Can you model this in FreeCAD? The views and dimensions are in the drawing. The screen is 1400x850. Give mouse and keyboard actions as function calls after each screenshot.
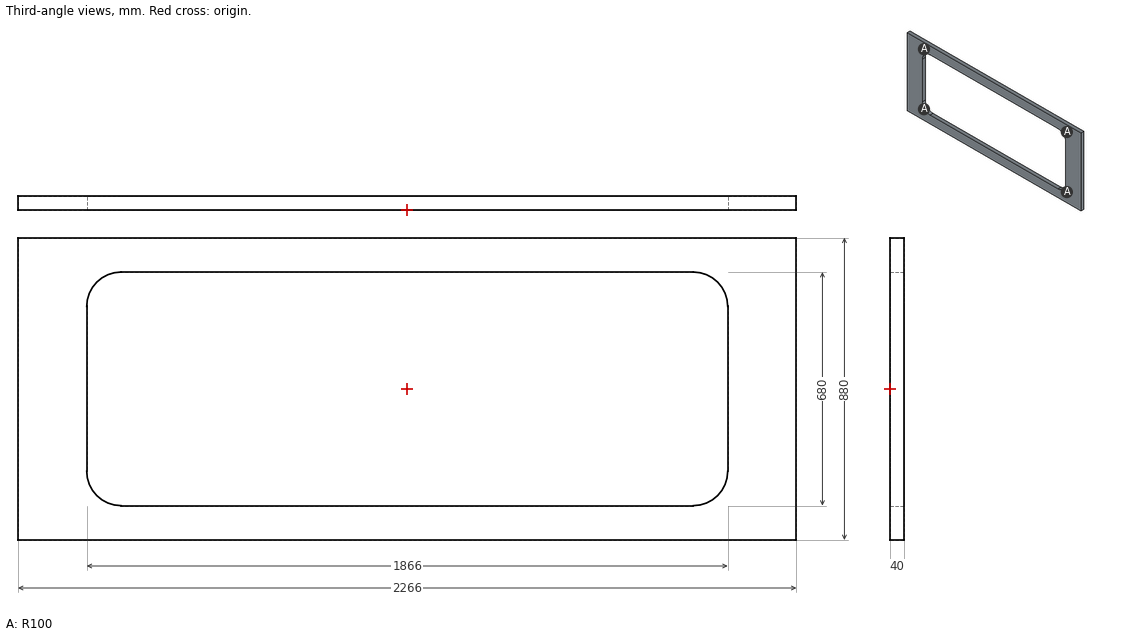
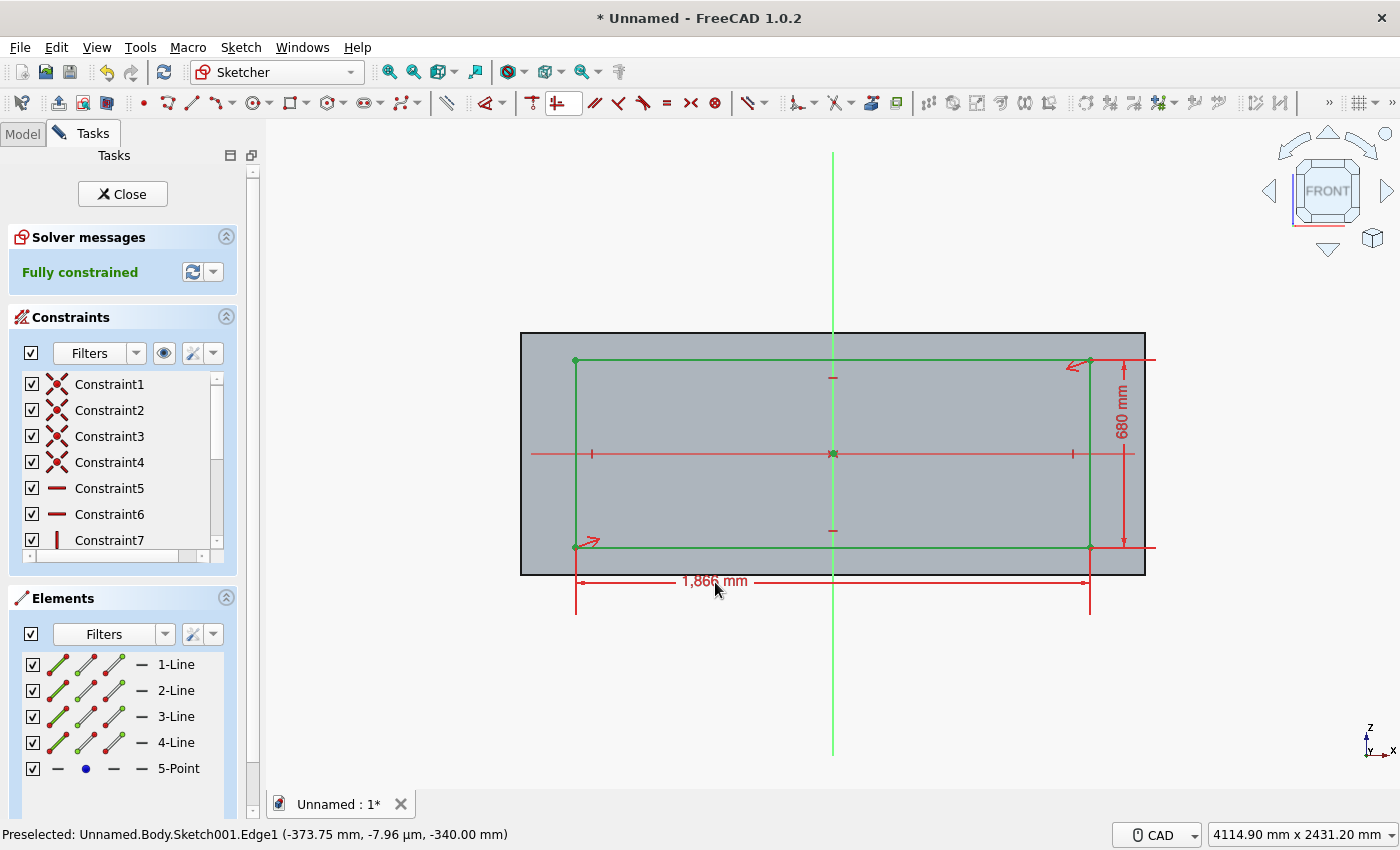
click(123, 194)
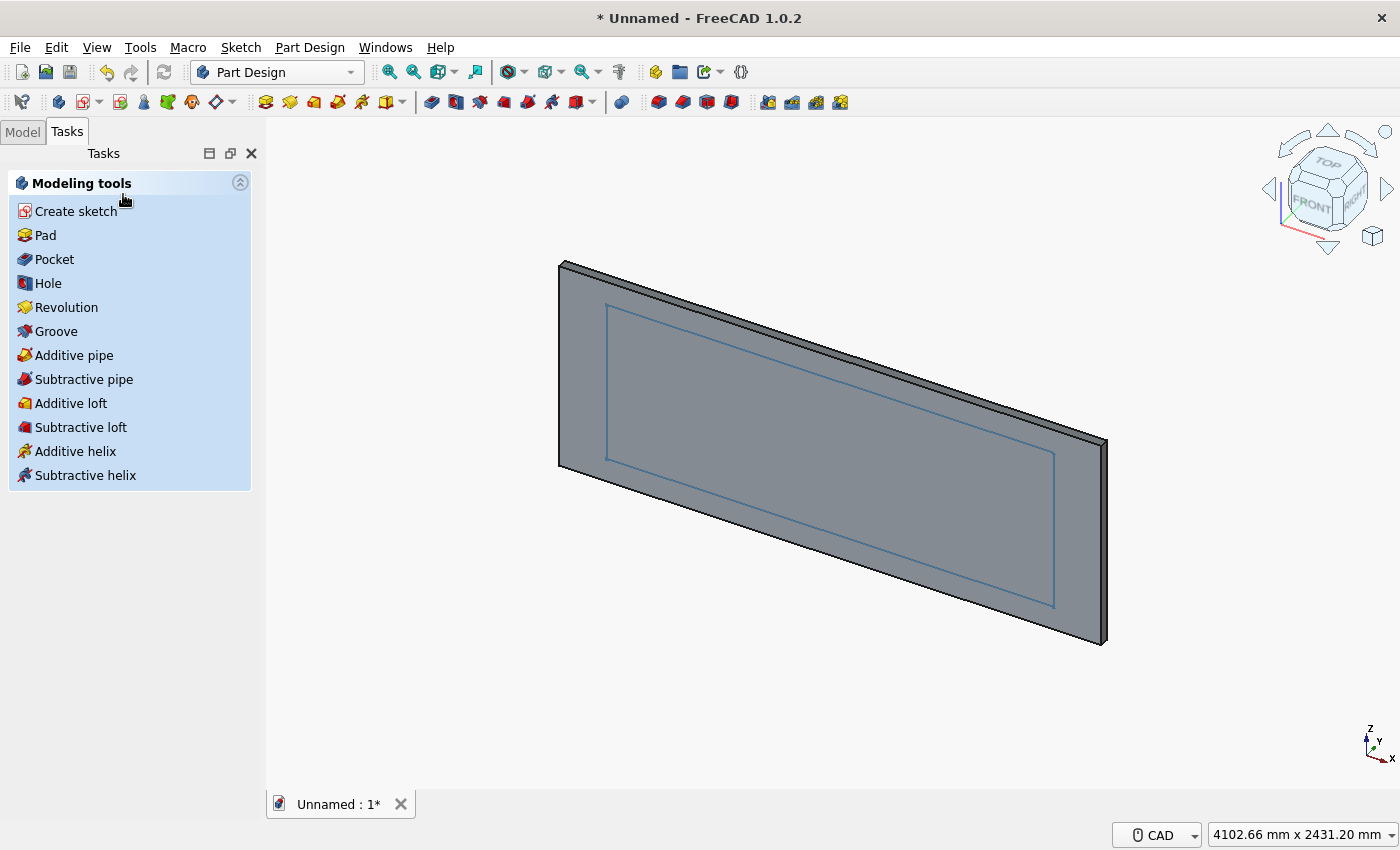
click(432, 102)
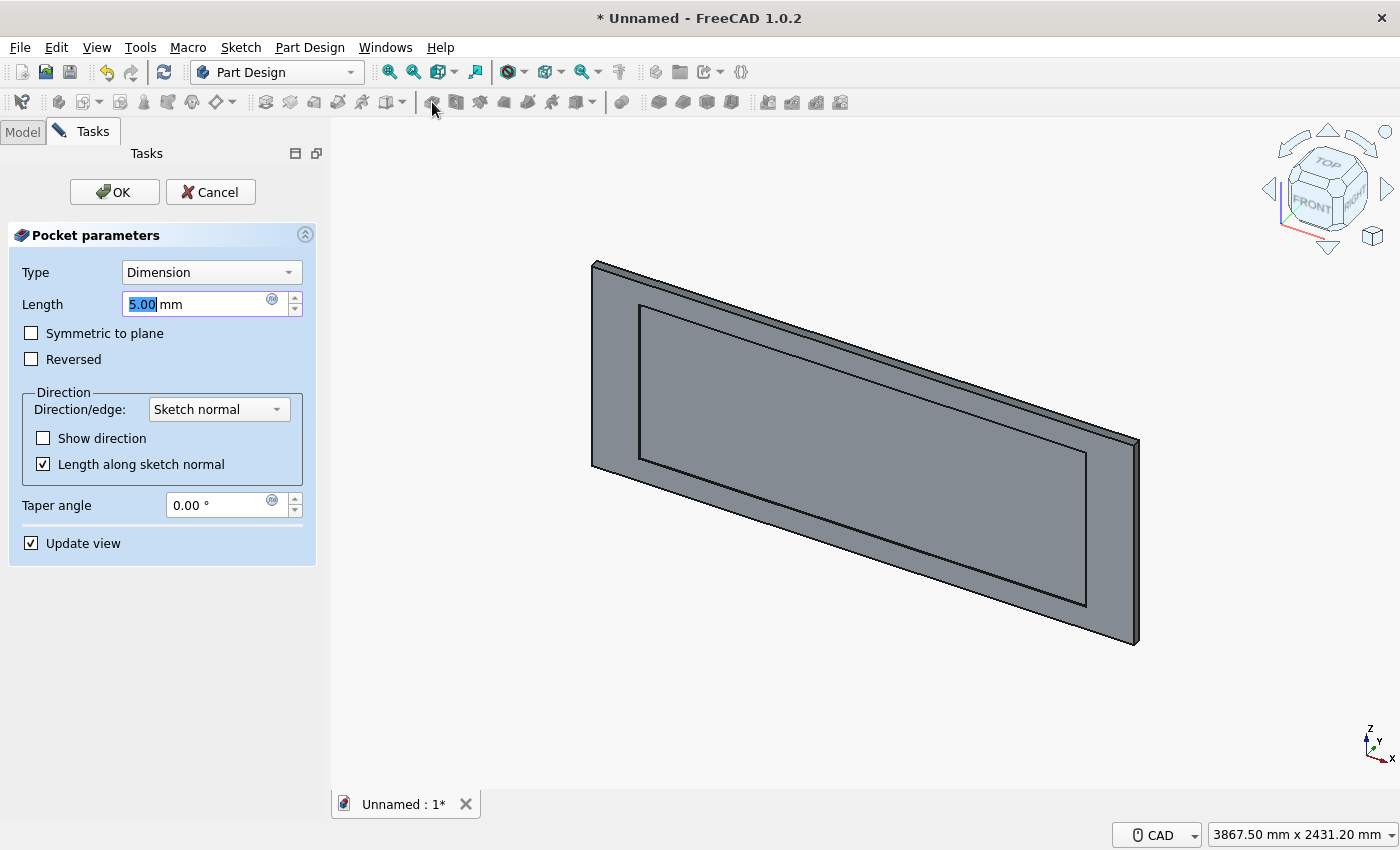
click(212, 272)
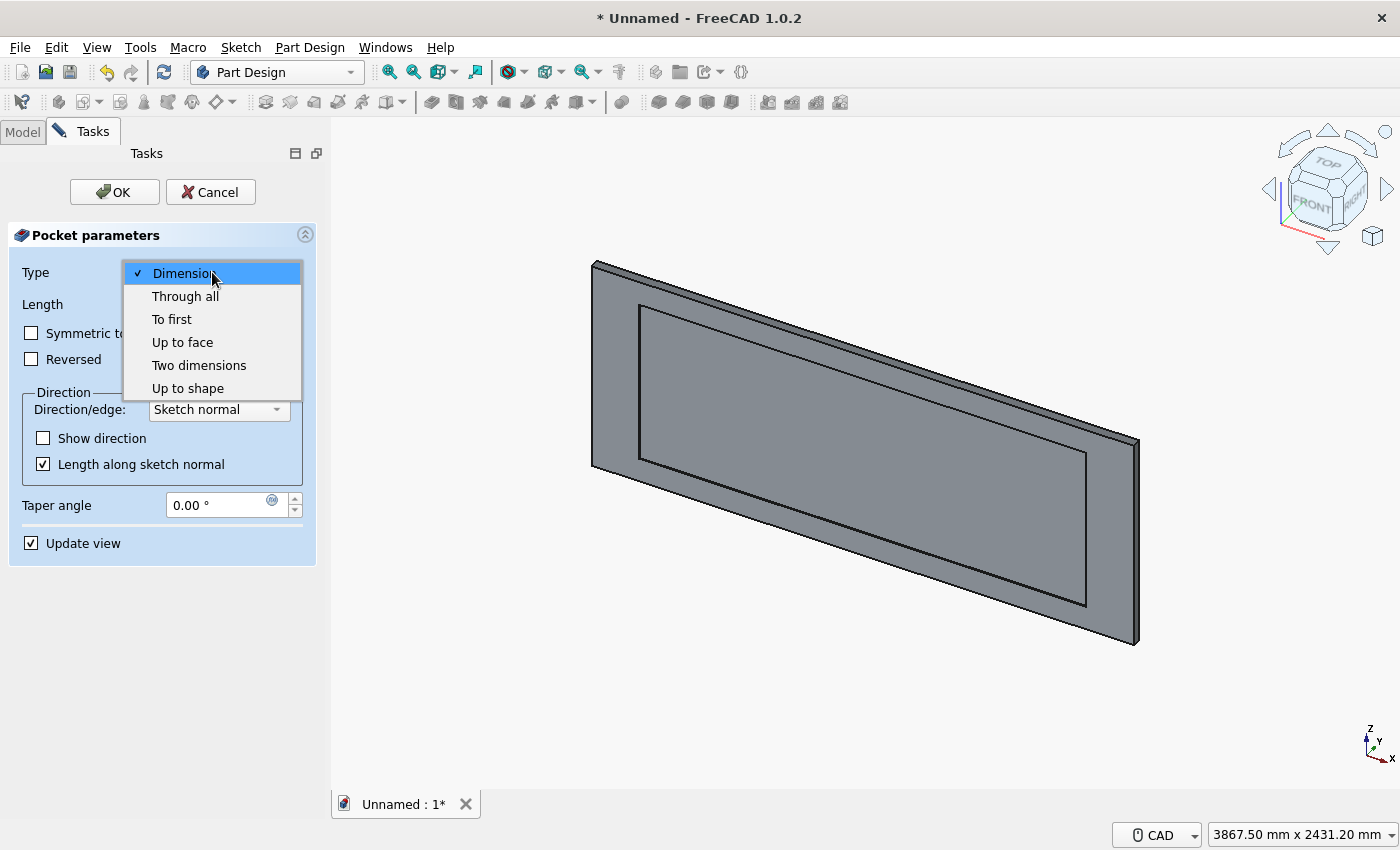
click(212, 296)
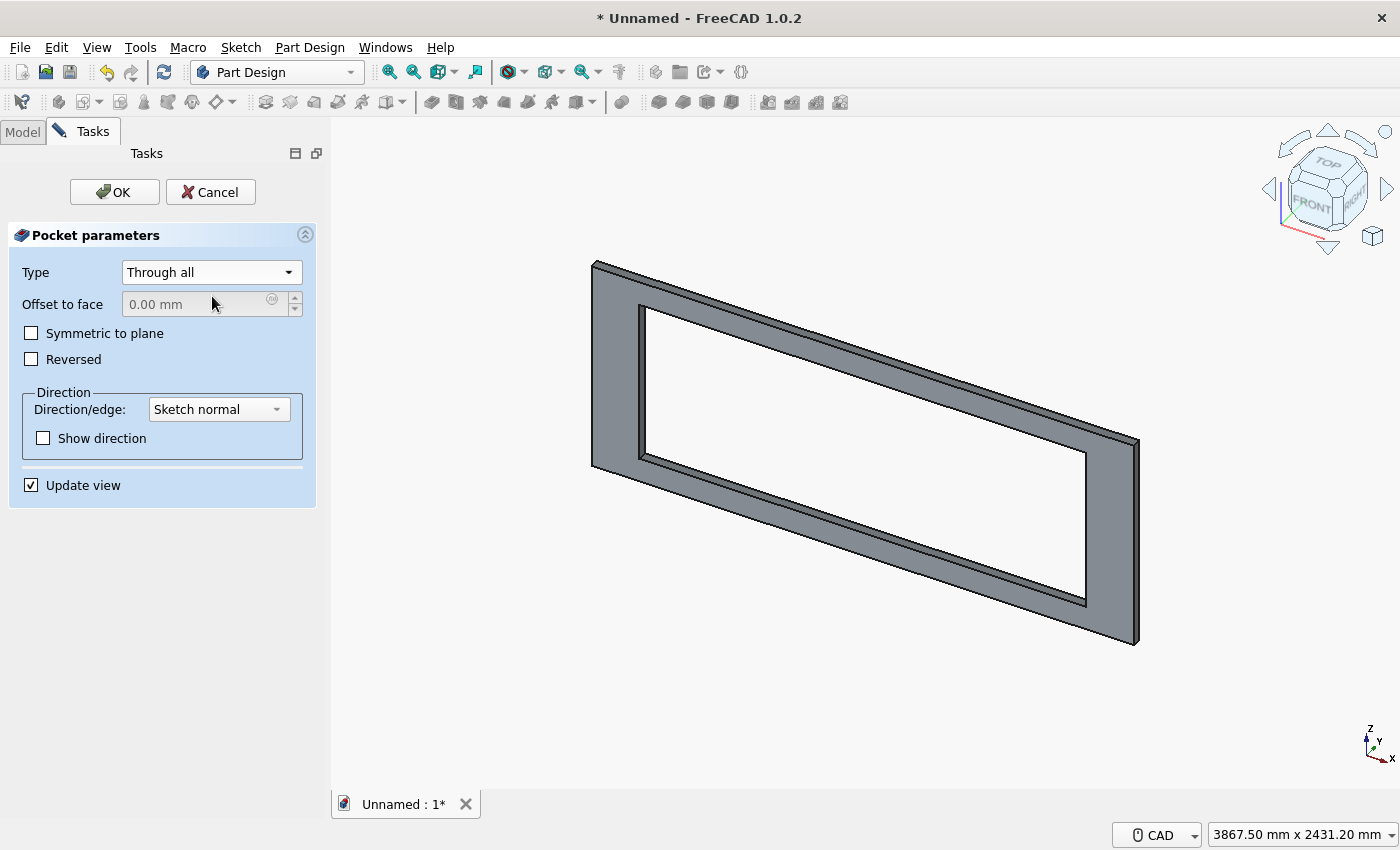
click(115, 192)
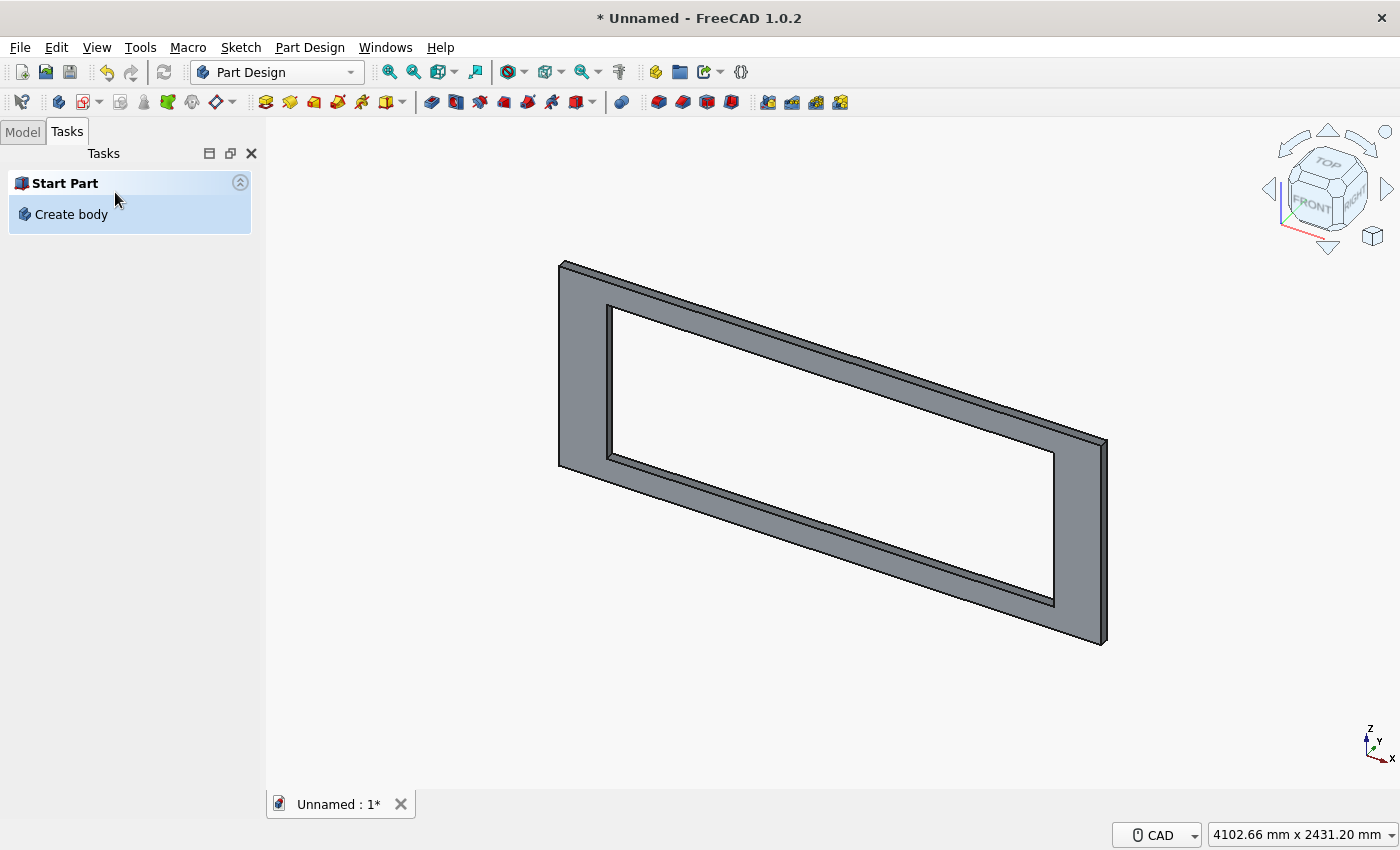
scroll(1056, 449, up, 7)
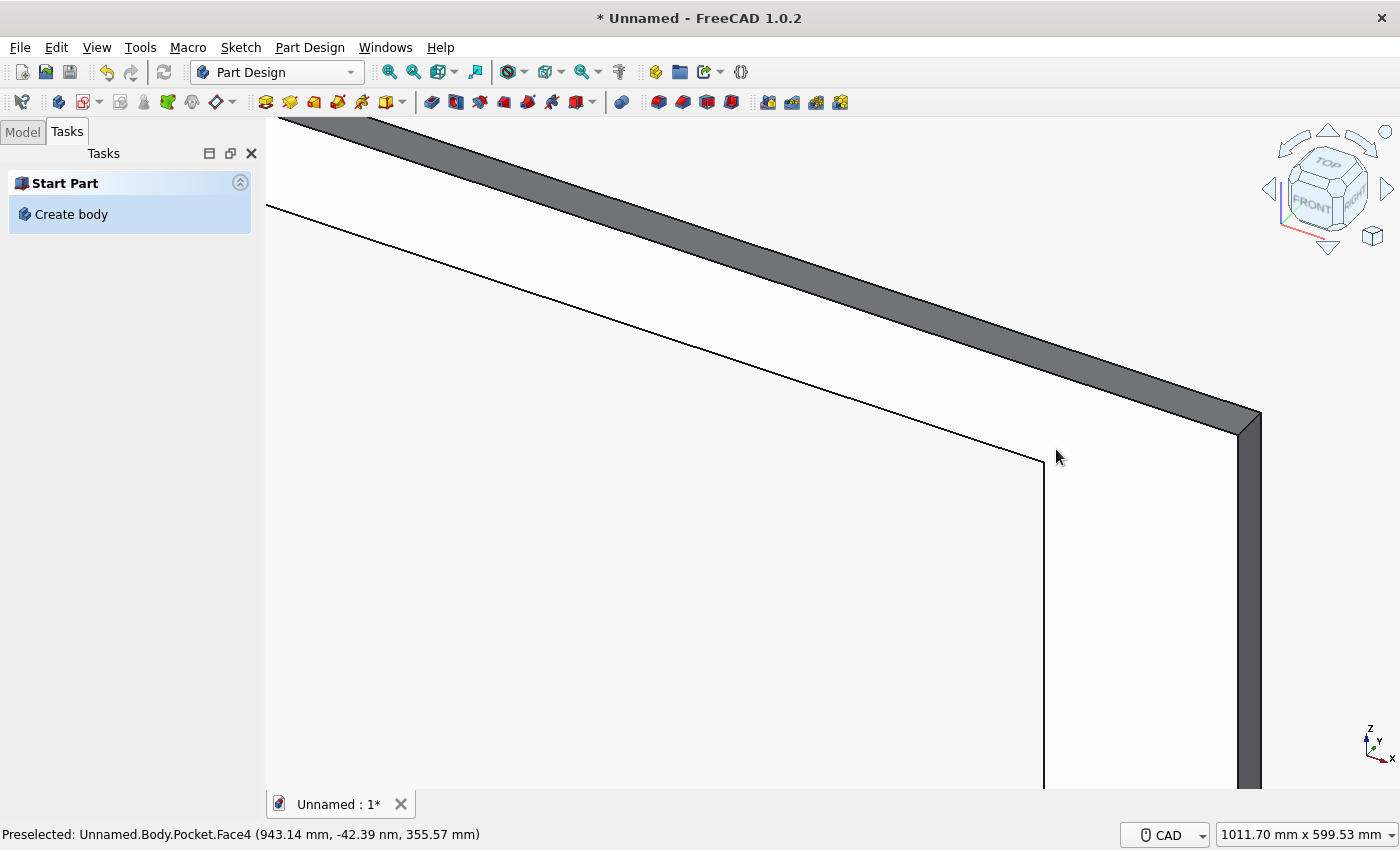
click(390, 72)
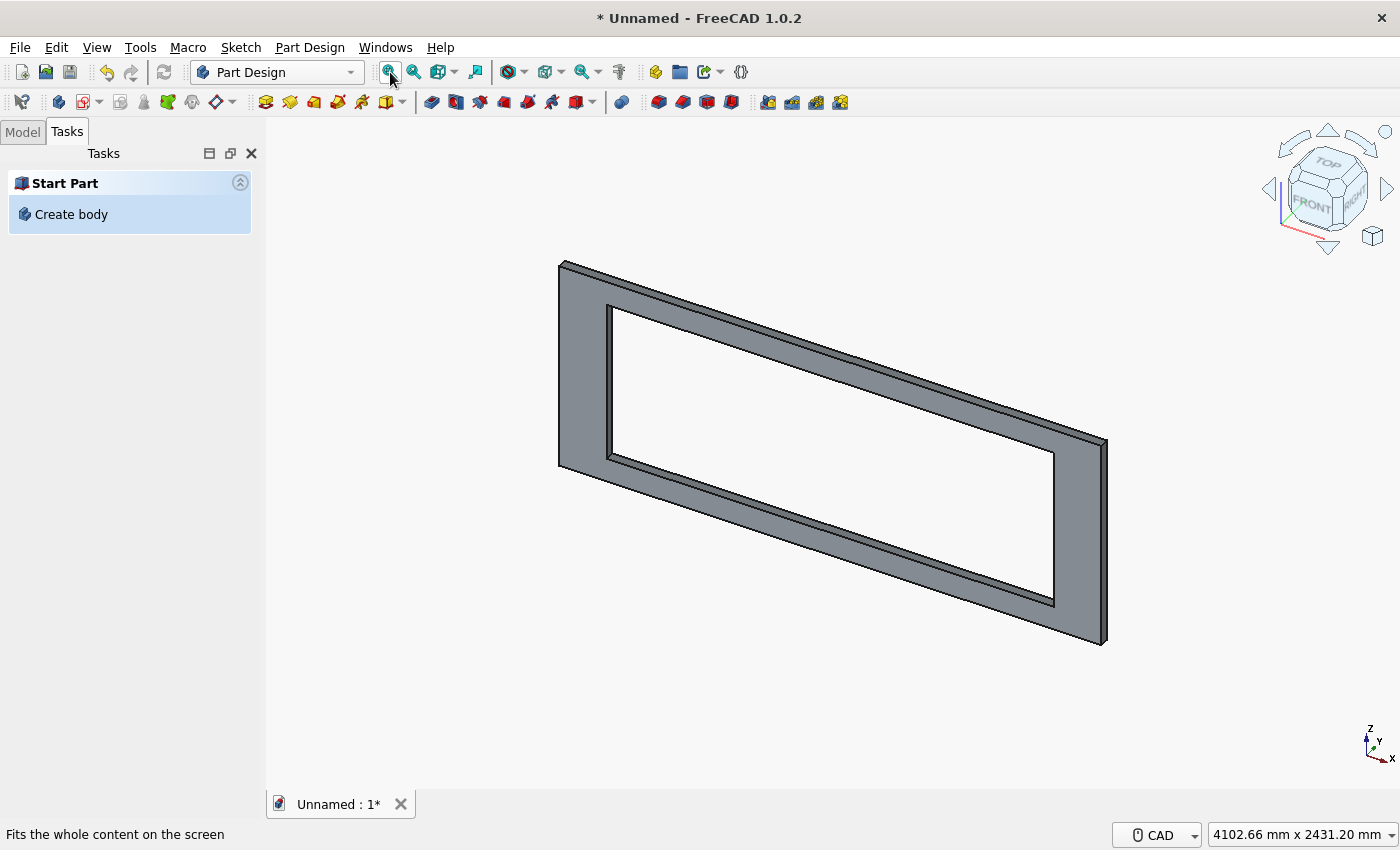
key(0)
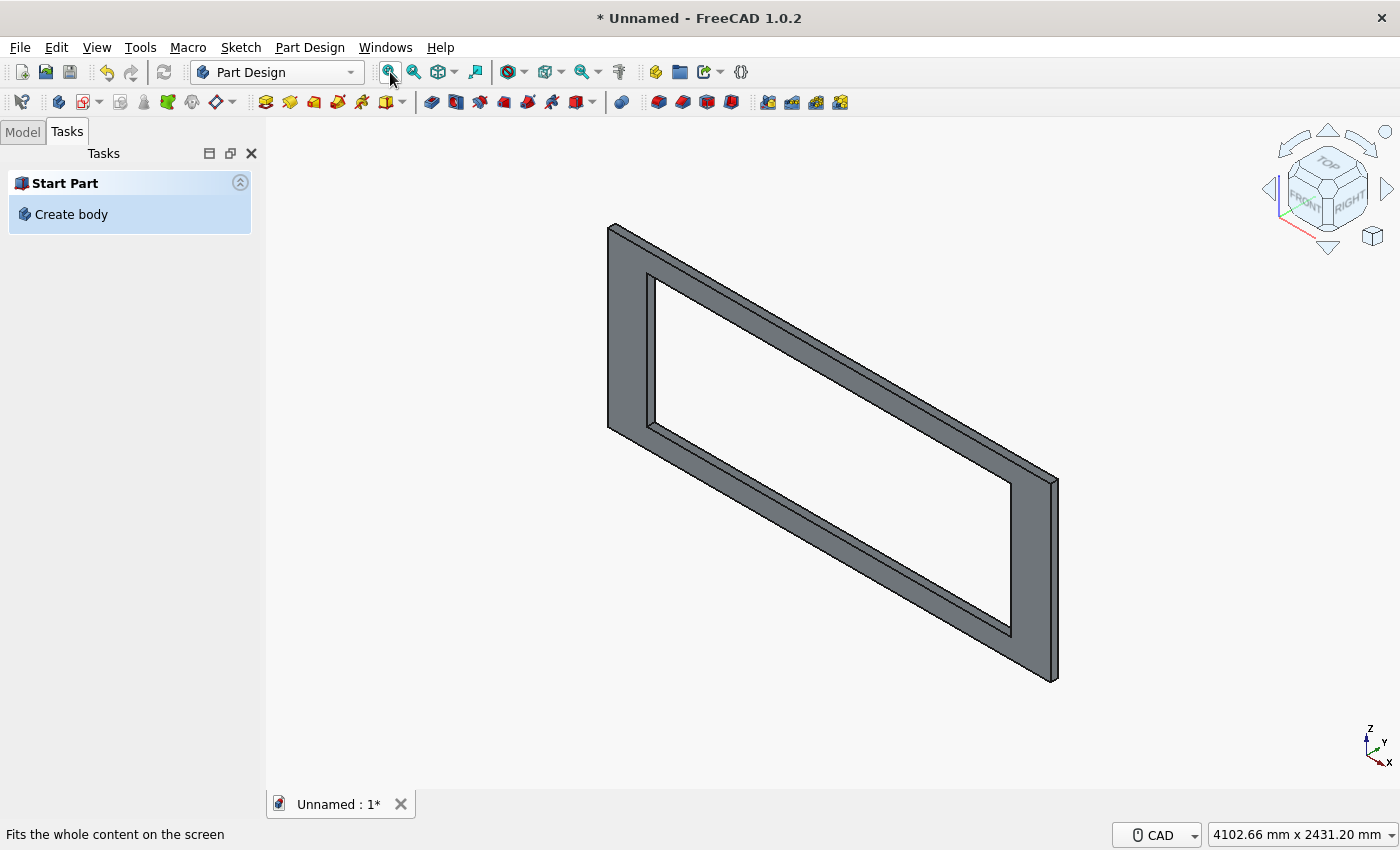
scroll(1015, 481, up, 7)